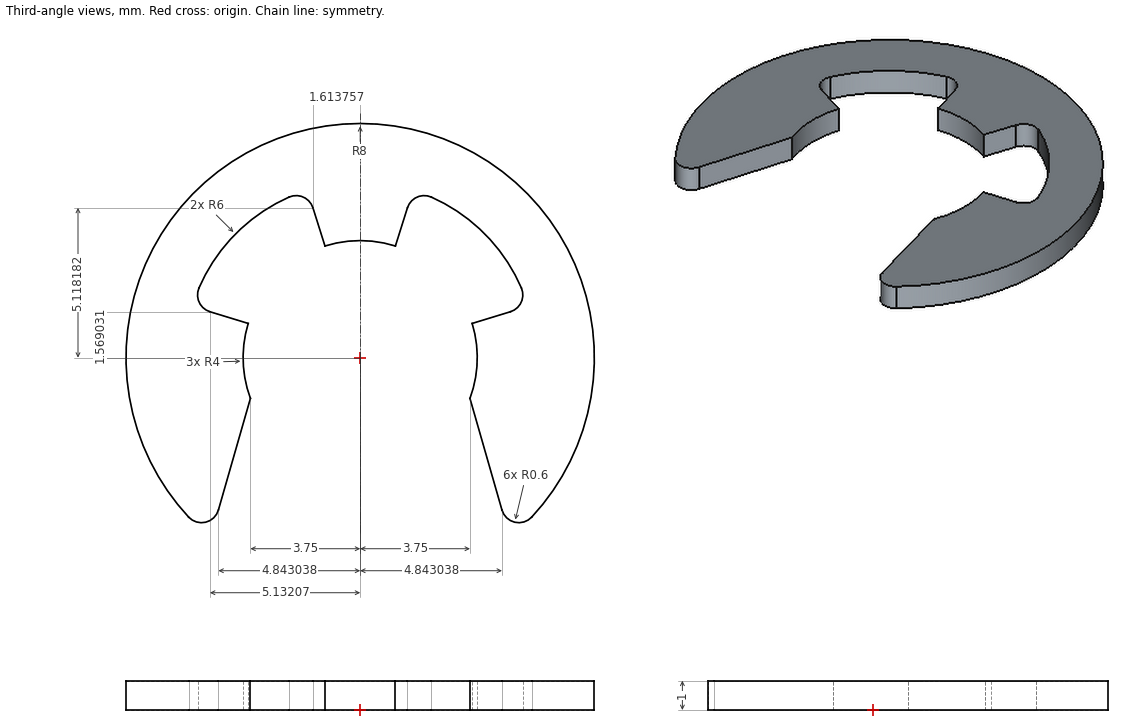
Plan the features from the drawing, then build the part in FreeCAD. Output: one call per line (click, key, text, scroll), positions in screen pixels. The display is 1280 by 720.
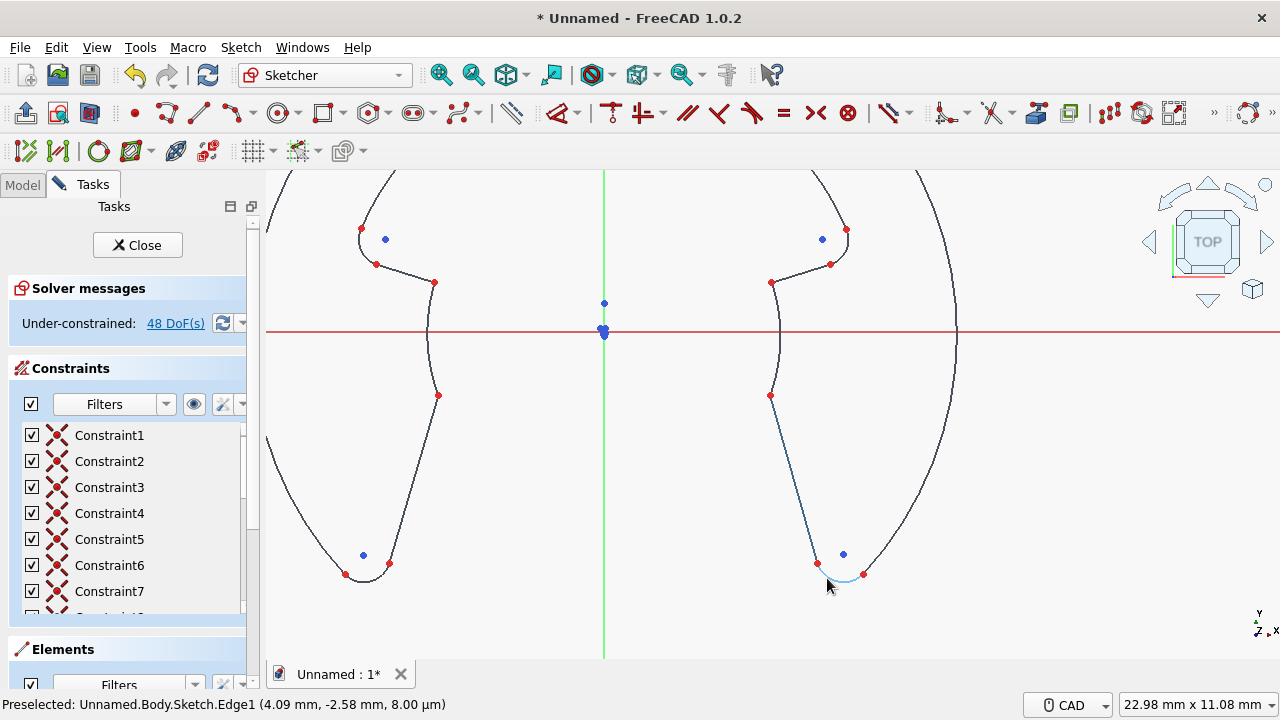
click(827, 577)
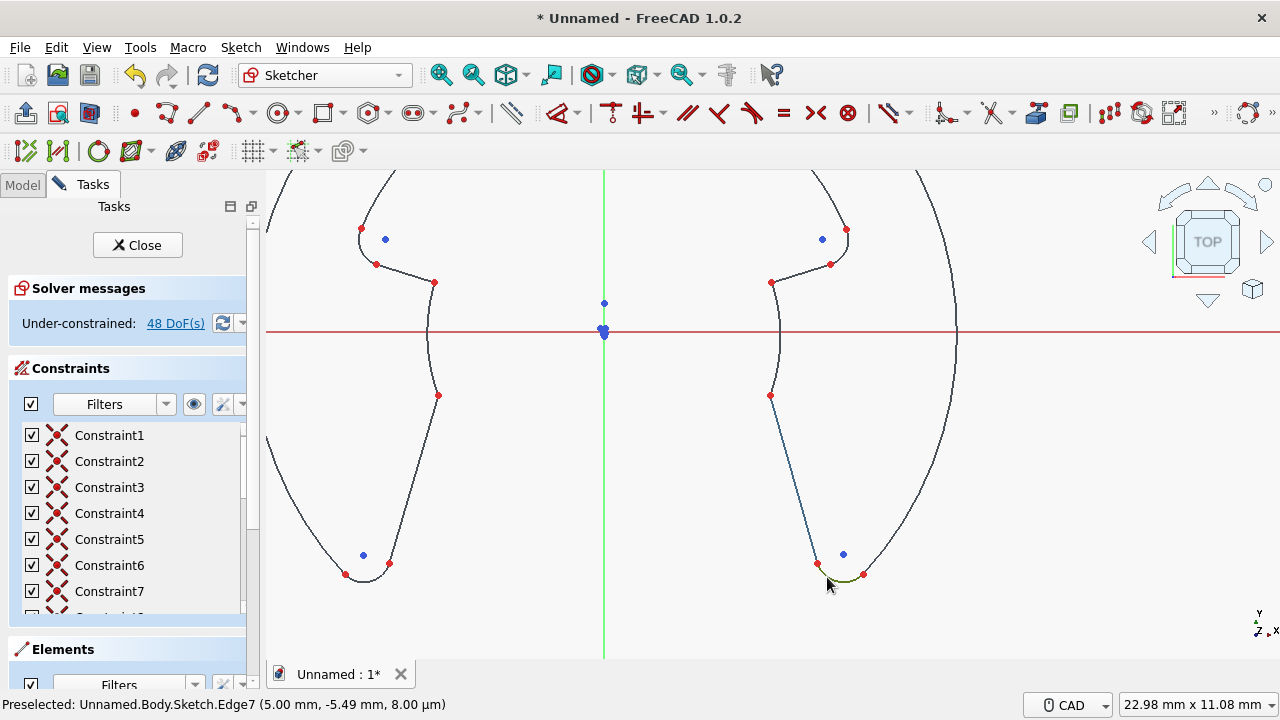
click(752, 114)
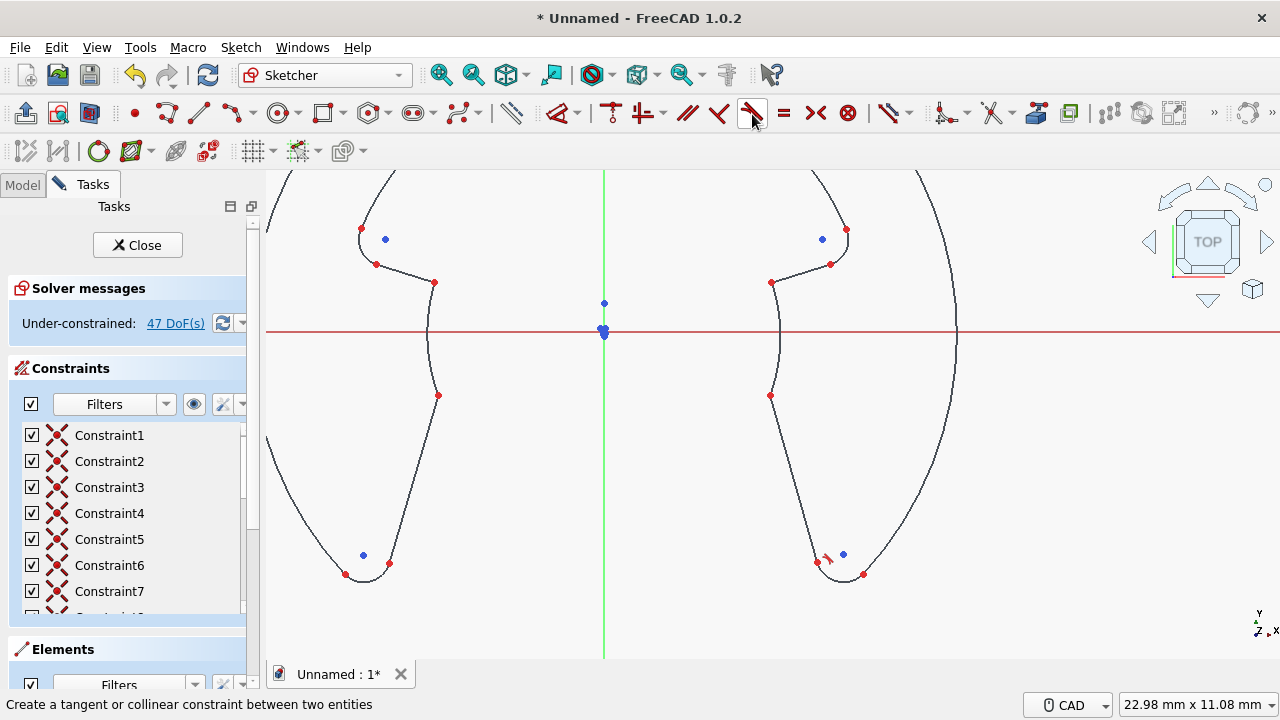
click(404, 513)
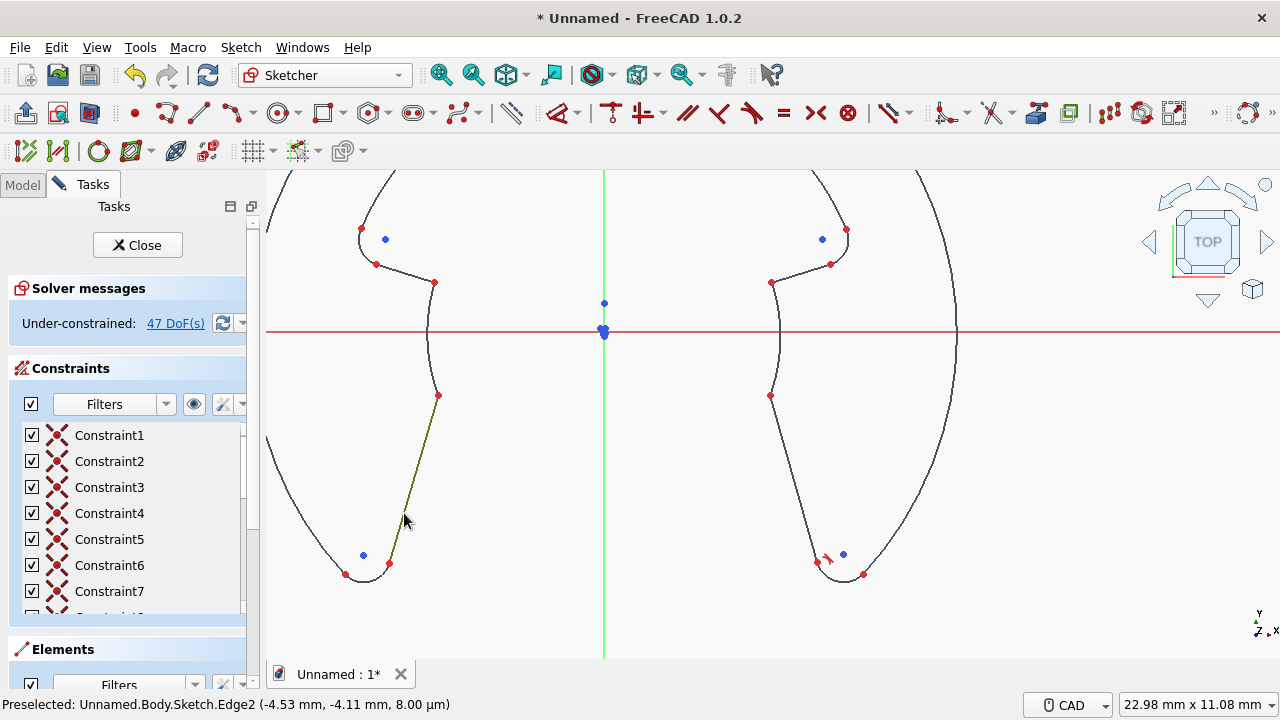
click(360, 582)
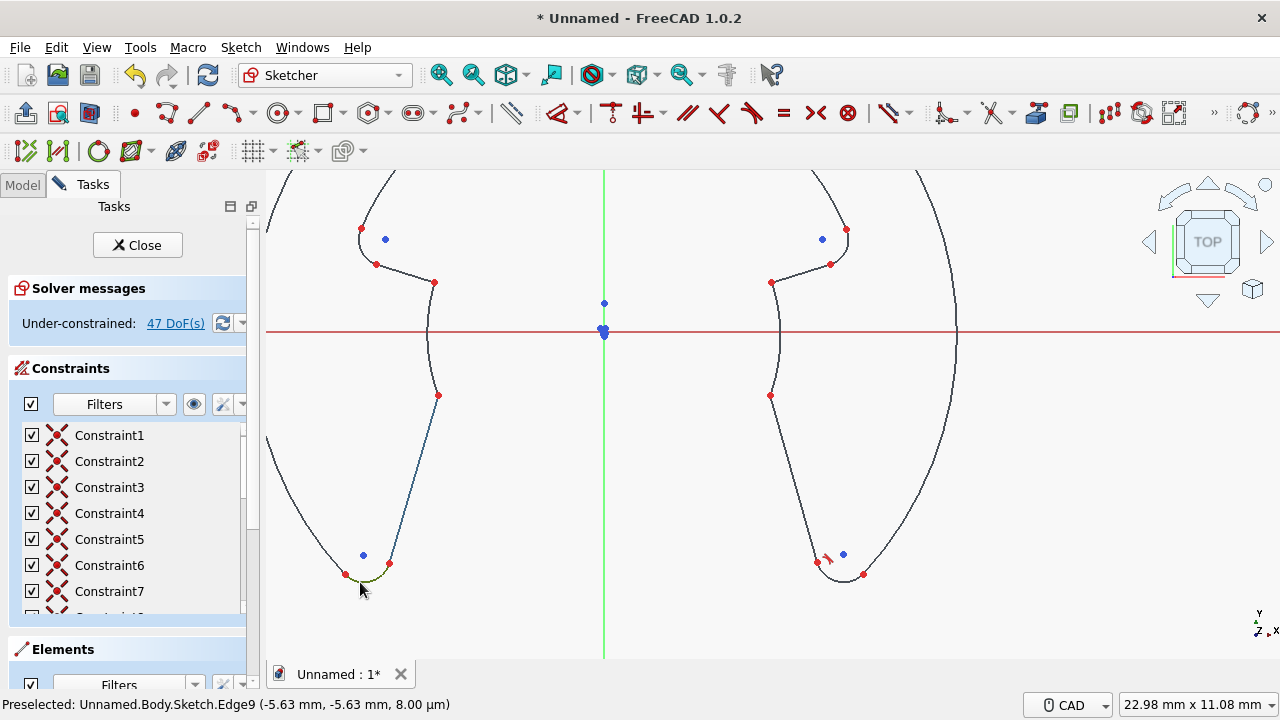
click(752, 114)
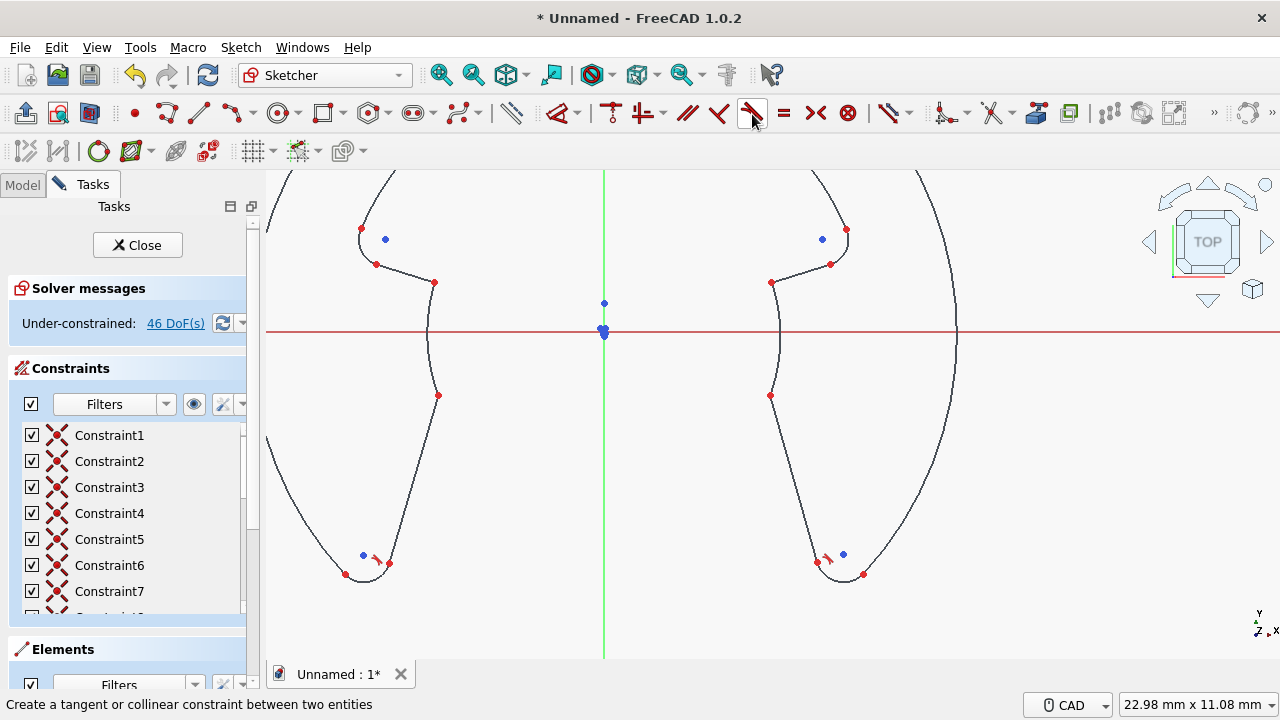
click(417, 277)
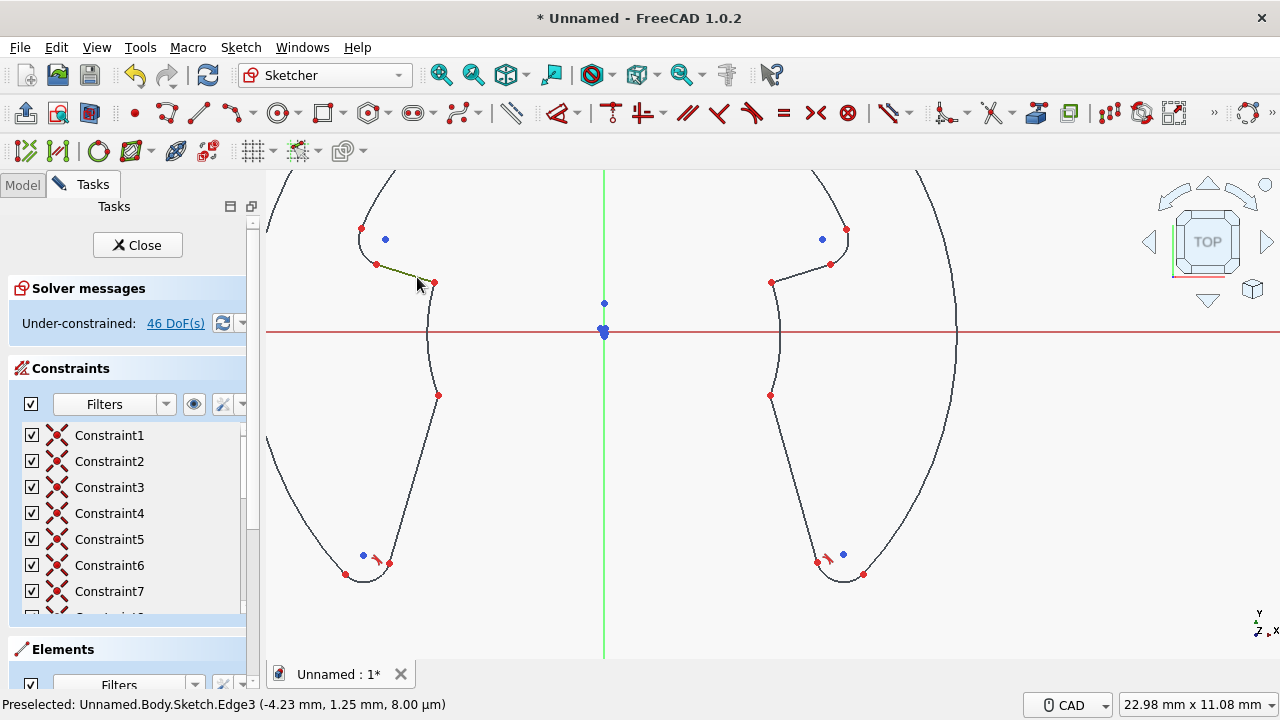
click(359, 241)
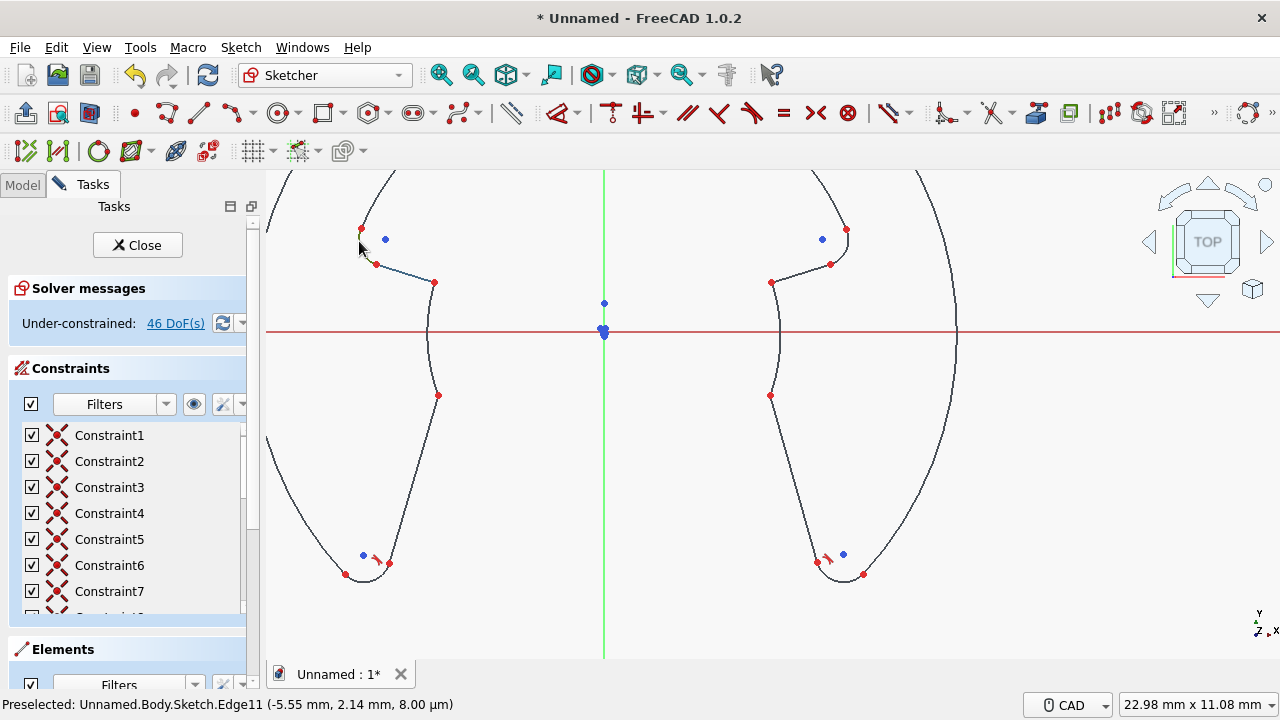
click(752, 114)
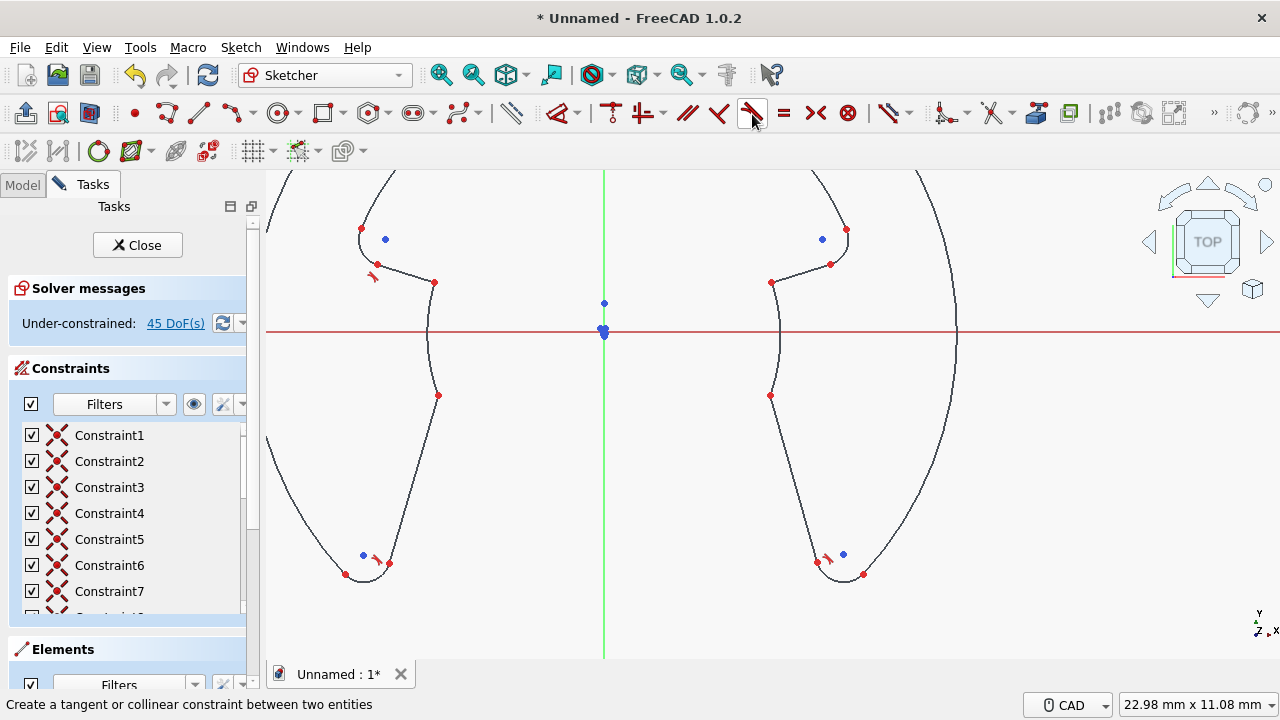
scroll(827, 578, down, 3)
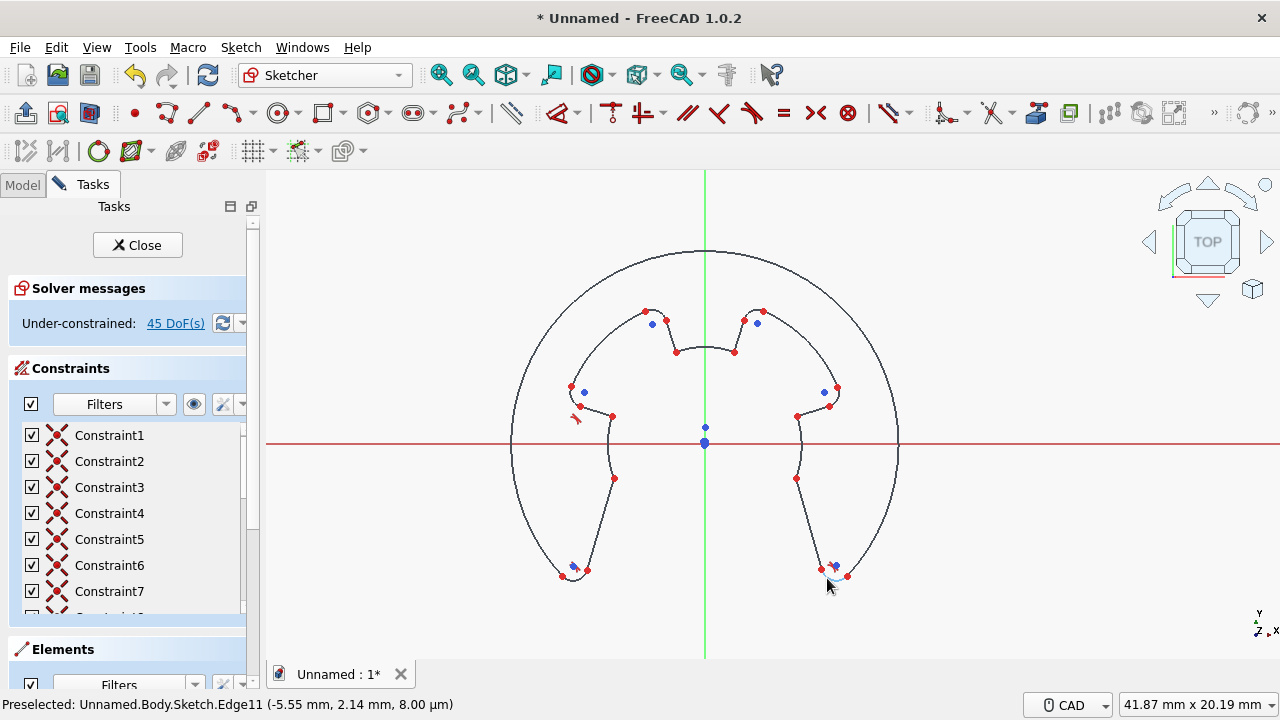
scroll(669, 330, up, 2)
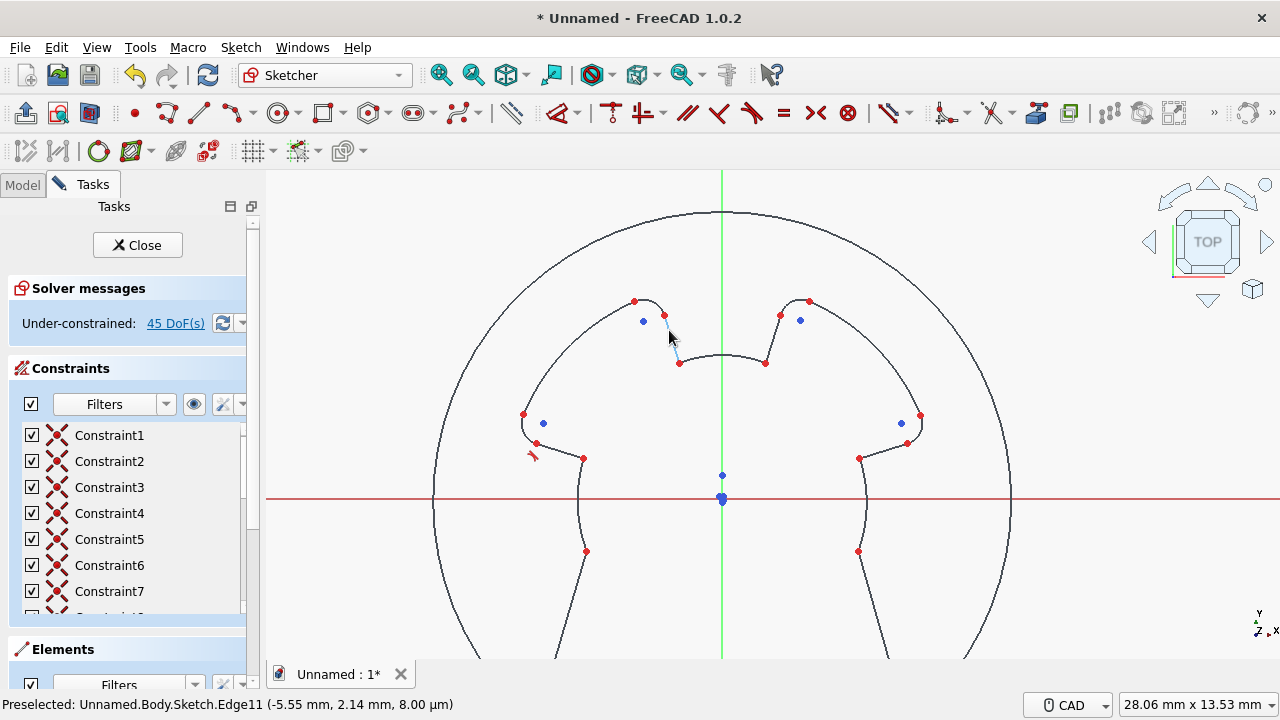
click(669, 330)